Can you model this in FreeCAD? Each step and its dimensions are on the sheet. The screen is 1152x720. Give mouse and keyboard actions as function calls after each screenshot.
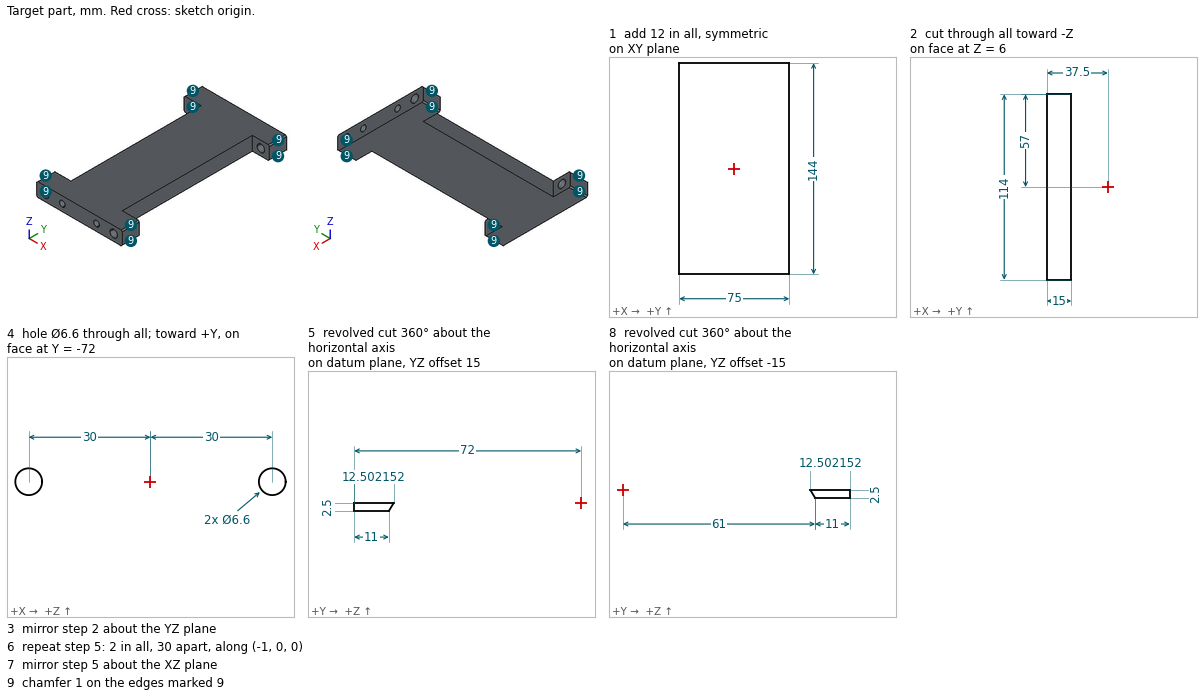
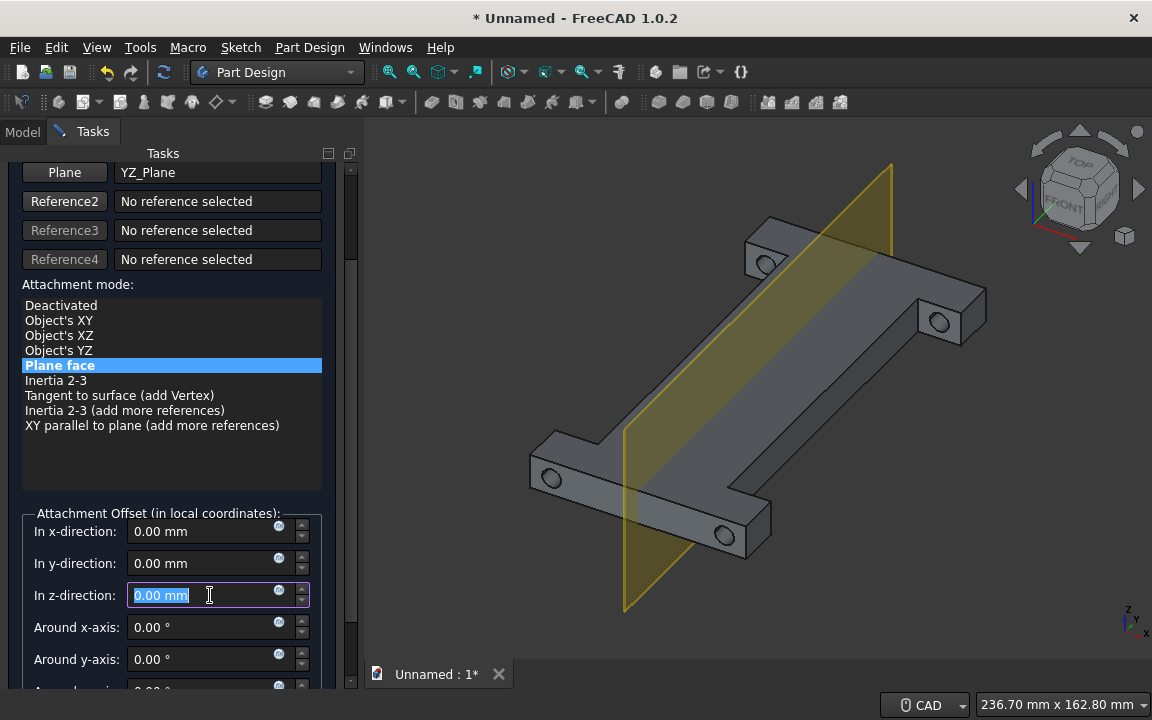
text(15)
key(Tab)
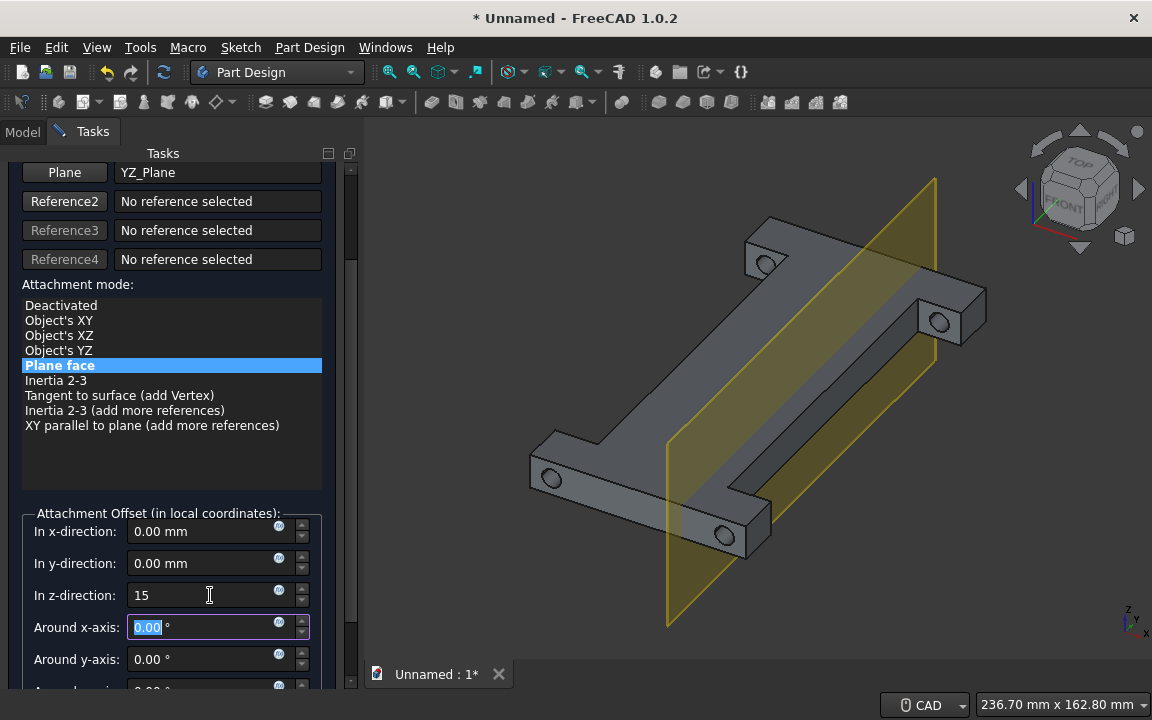
scroll(351, 426, up, 3)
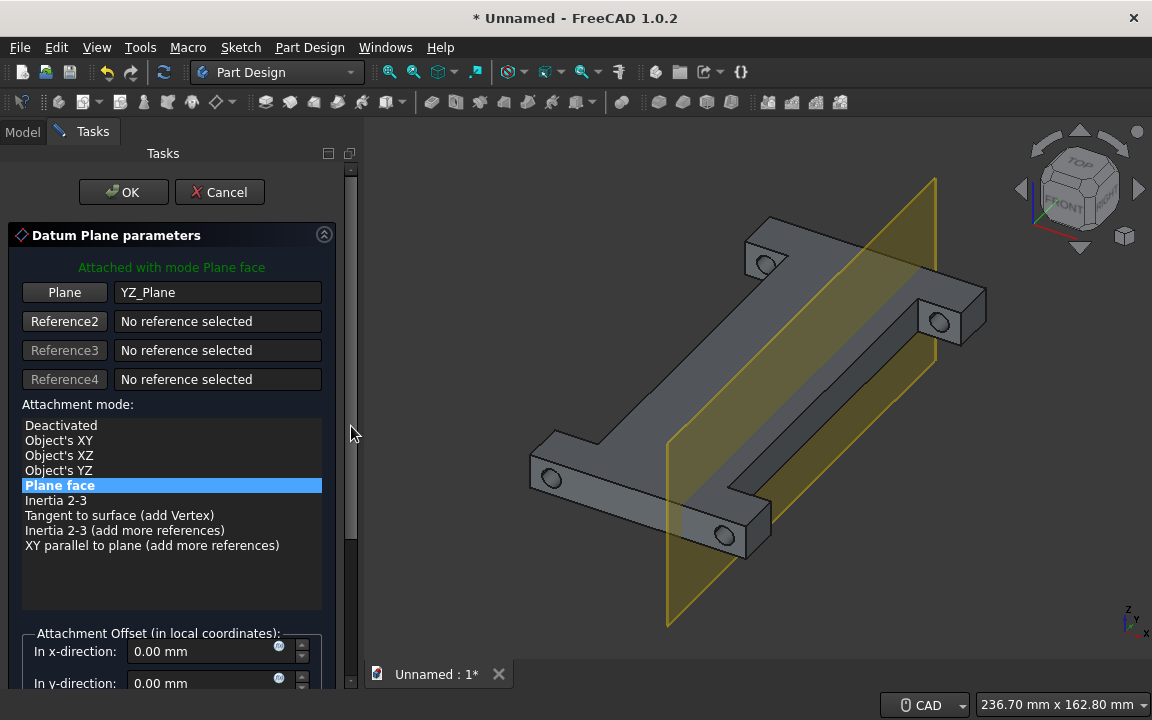
click(124, 192)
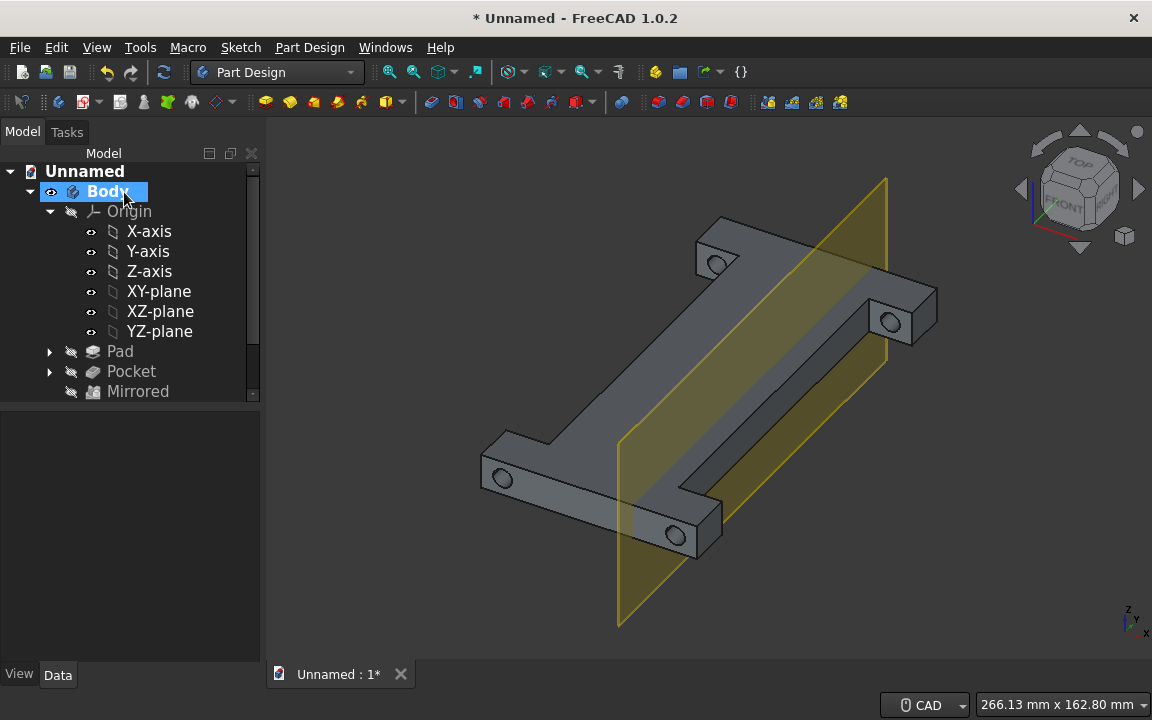
scroll(100, 287, down, 3)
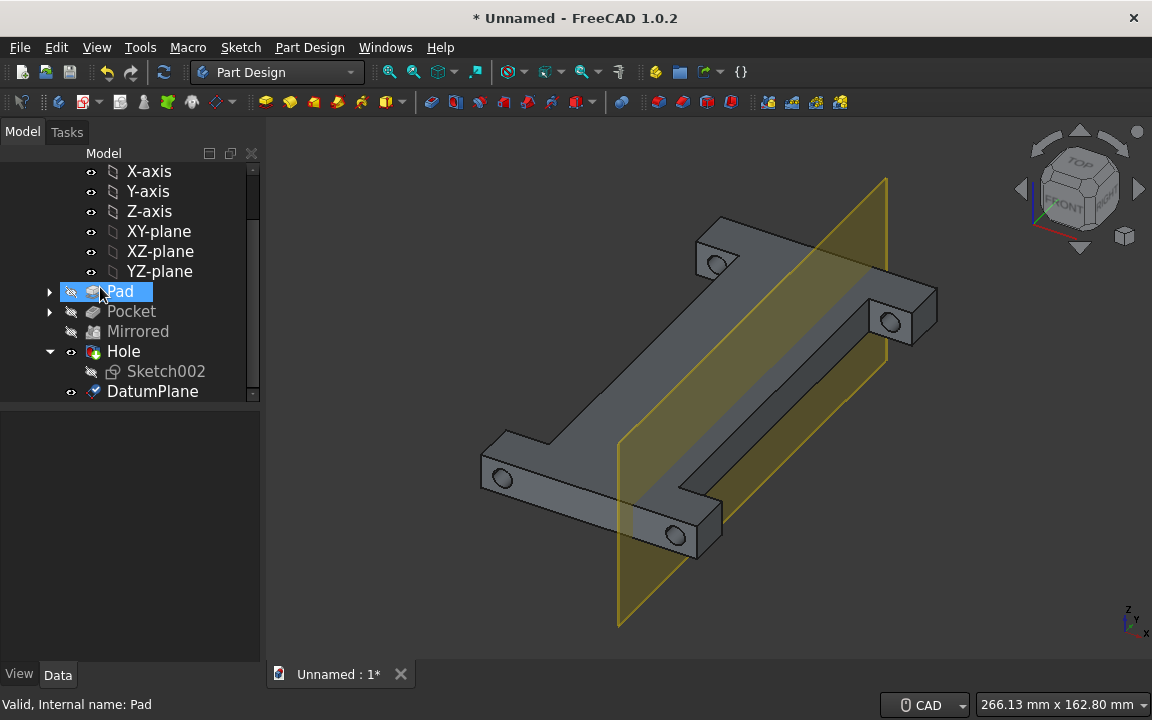
click(116, 392)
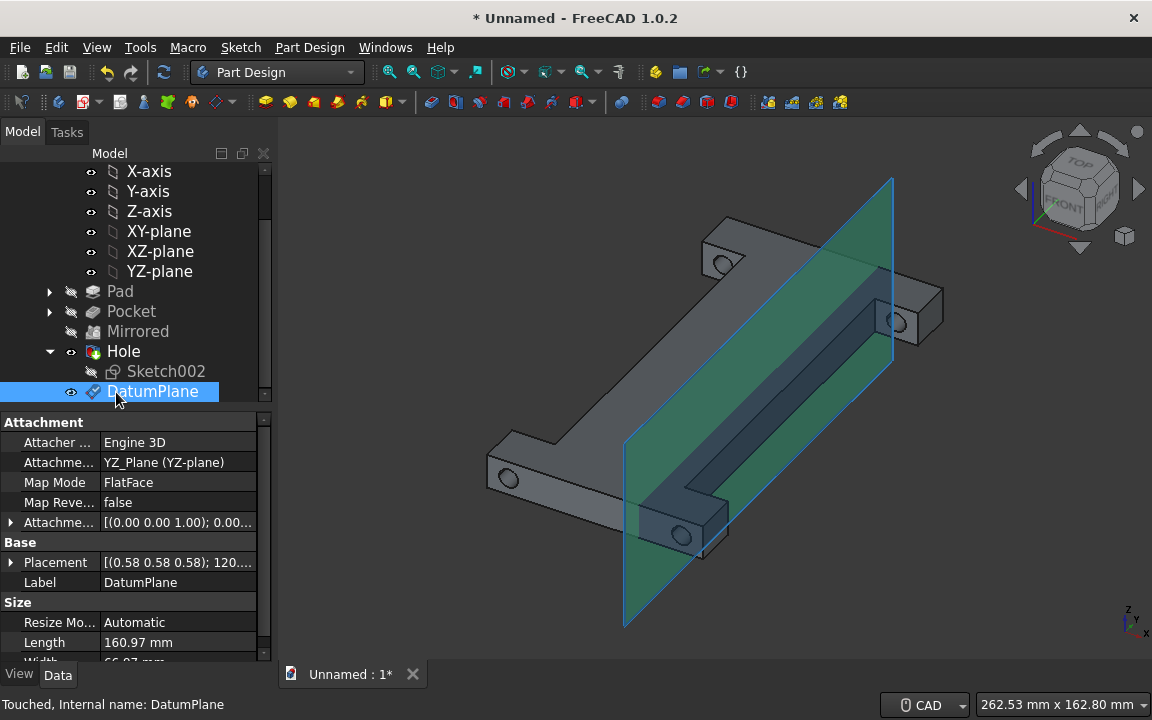
click(84, 102)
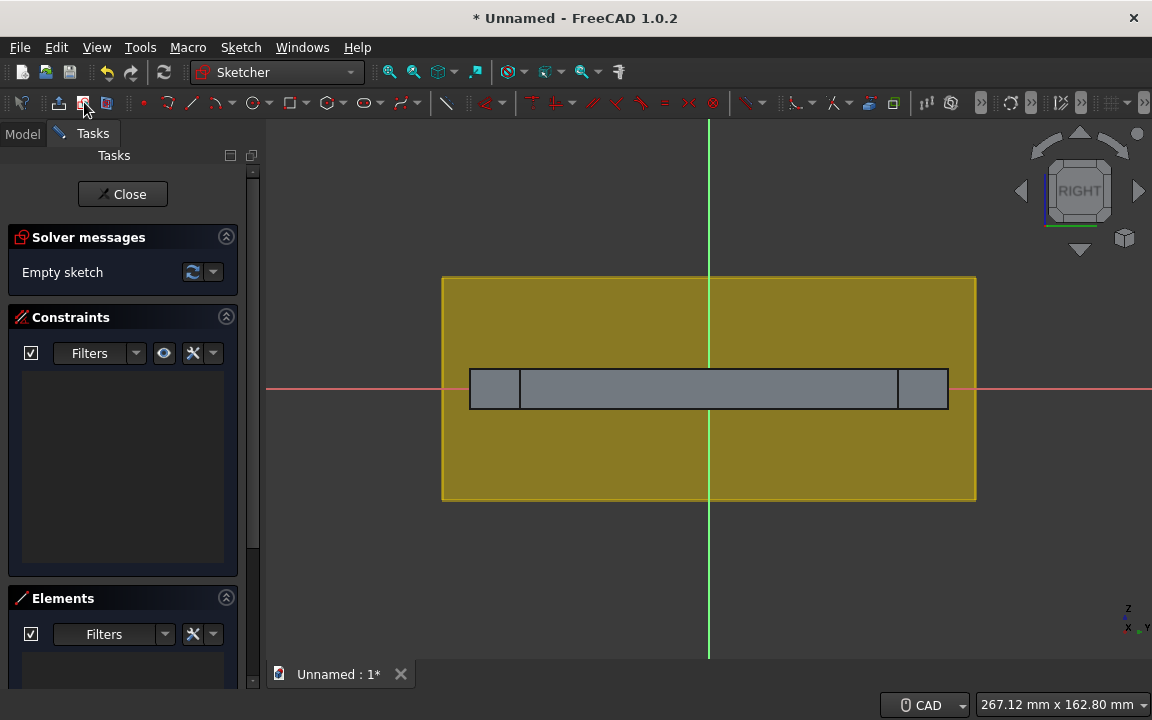
click(108, 104)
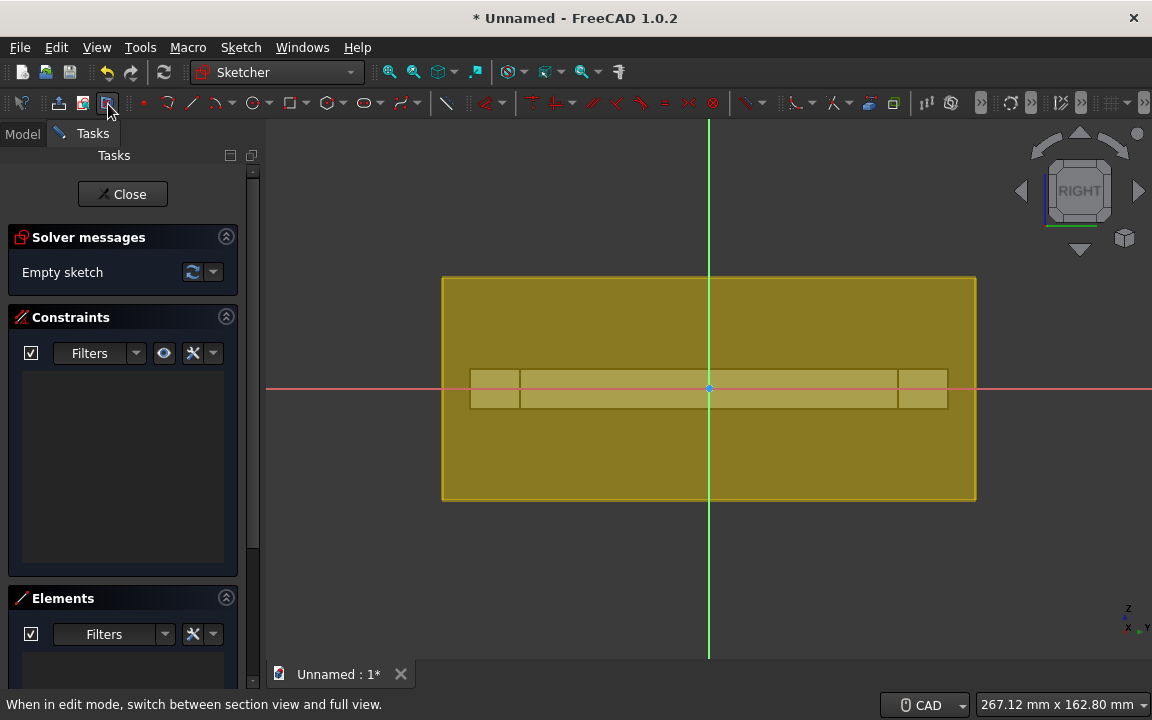
scroll(476, 394, up, 12)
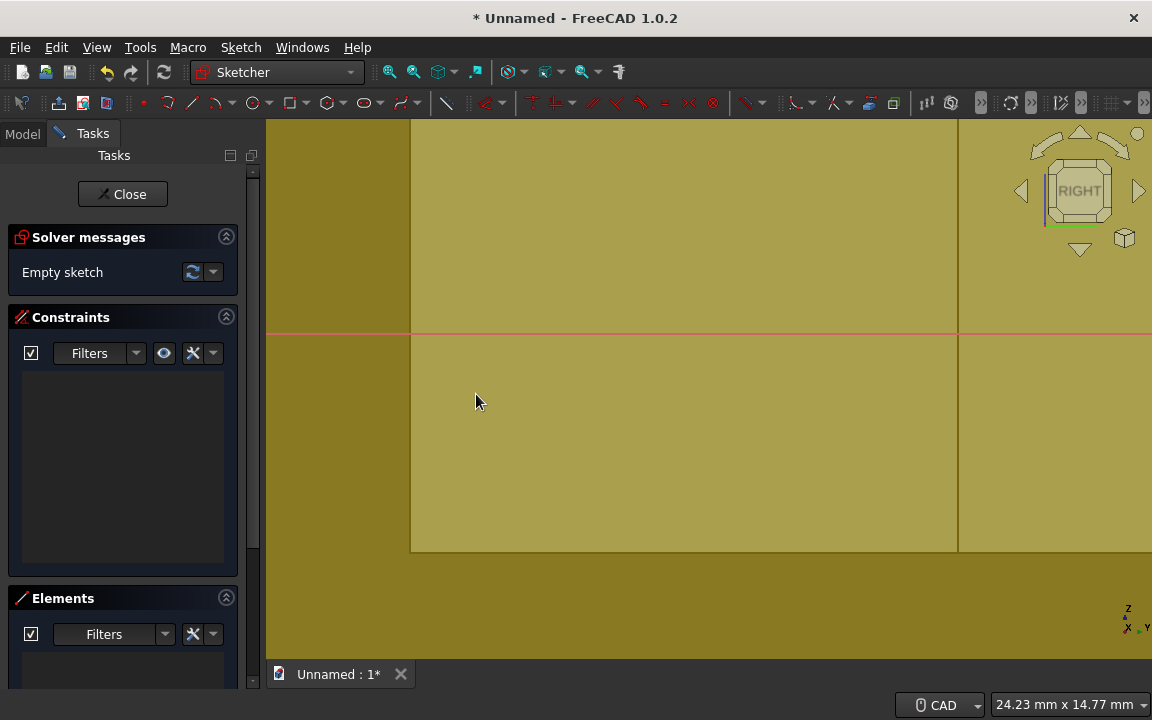
click(168, 104)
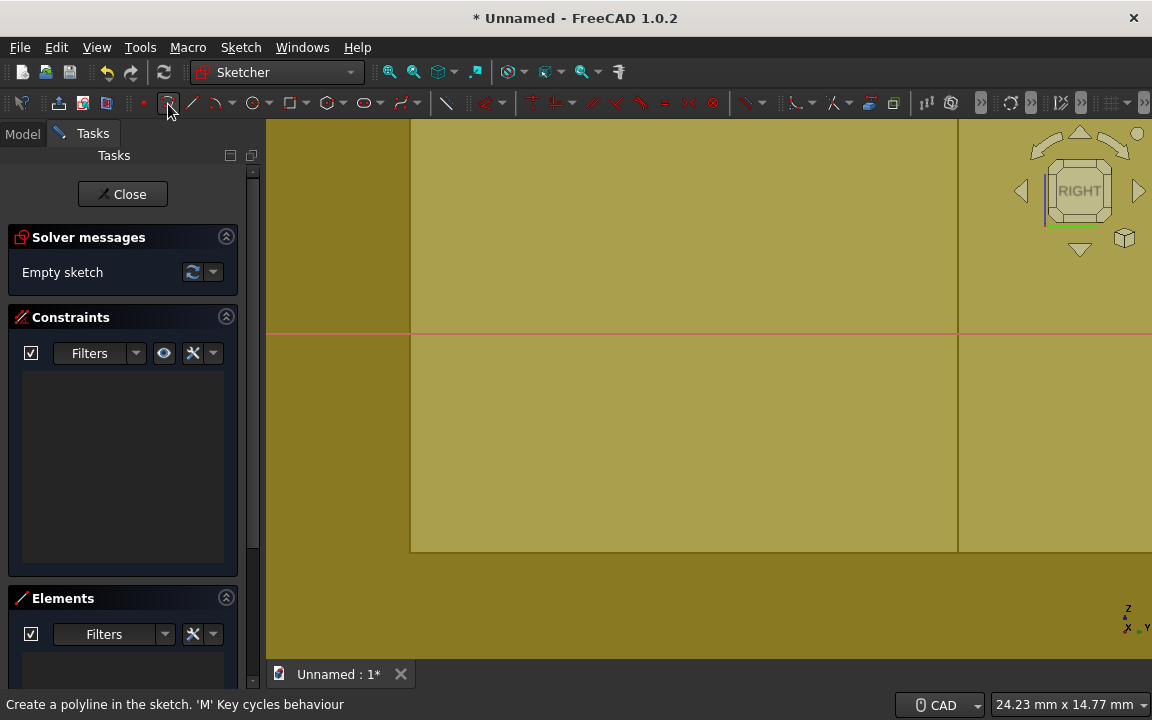
click(867, 334)
click(410, 343)
click(410, 425)
click(812, 425)
click(867, 334)
key(Escape)
key(Escape)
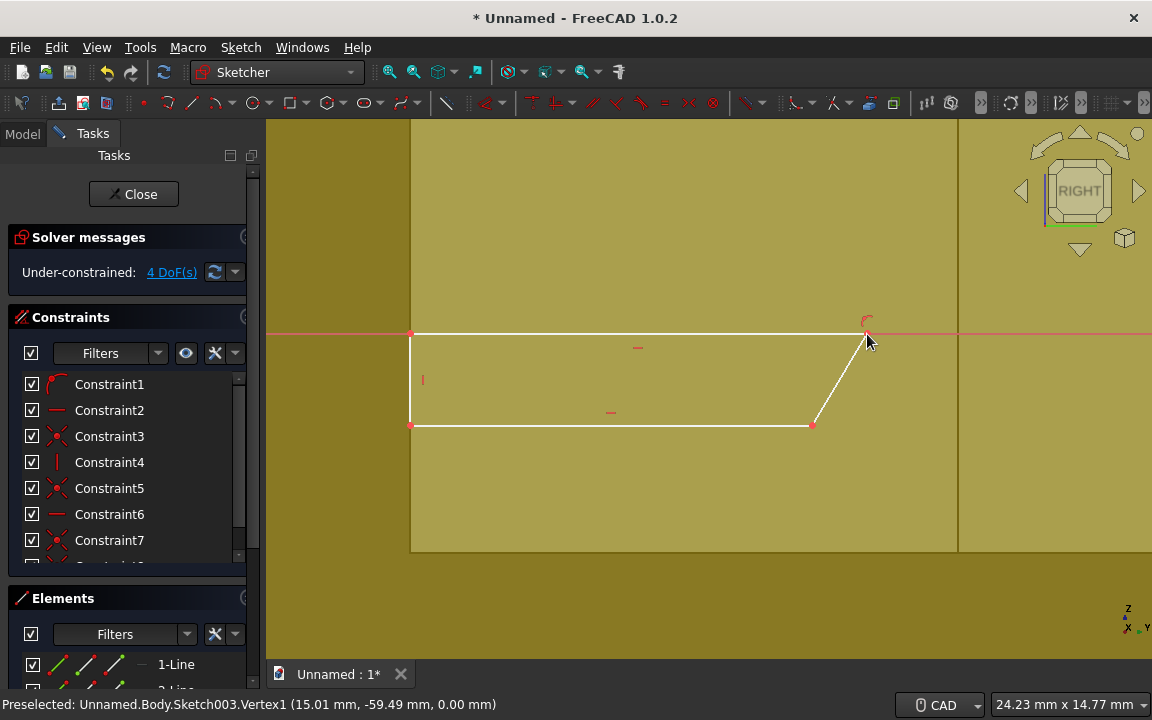
click(486, 104)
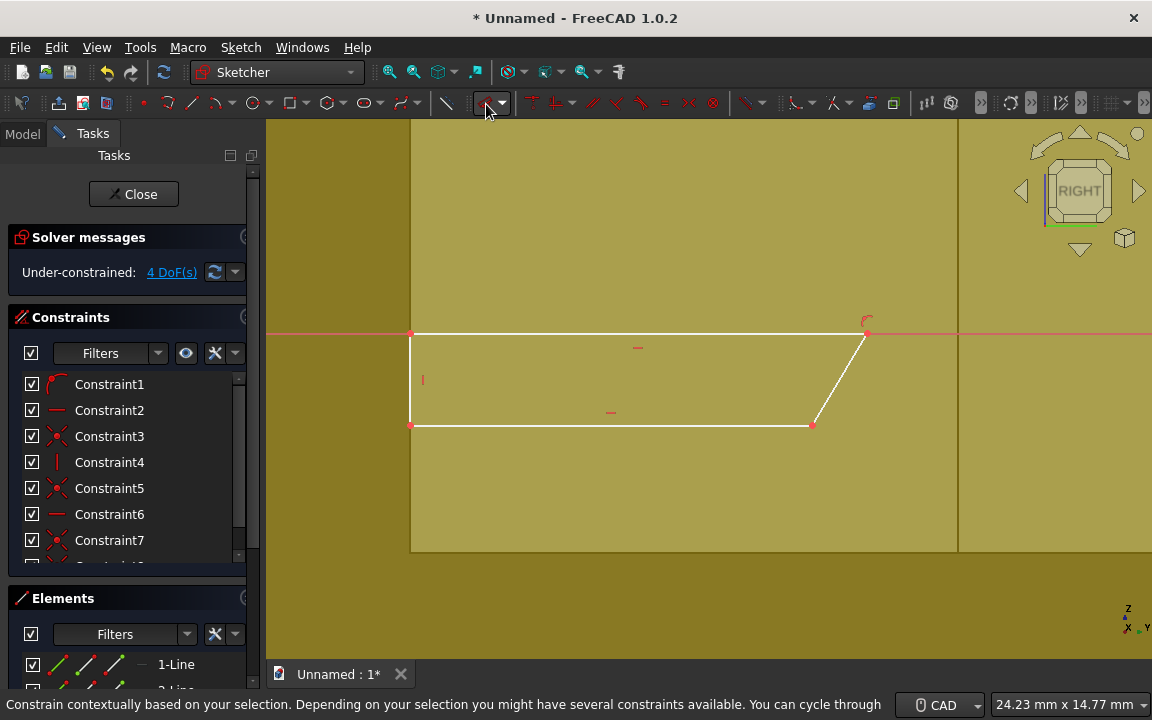
click(531, 426)
click(611, 460)